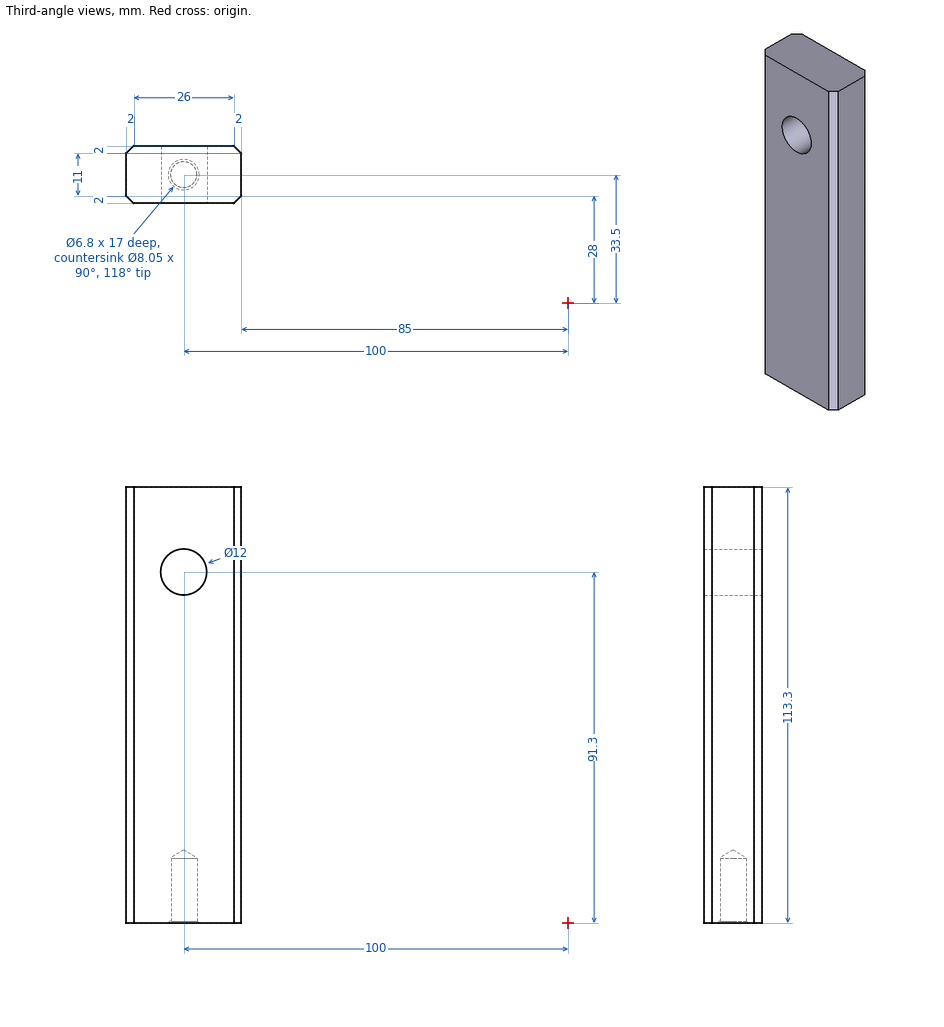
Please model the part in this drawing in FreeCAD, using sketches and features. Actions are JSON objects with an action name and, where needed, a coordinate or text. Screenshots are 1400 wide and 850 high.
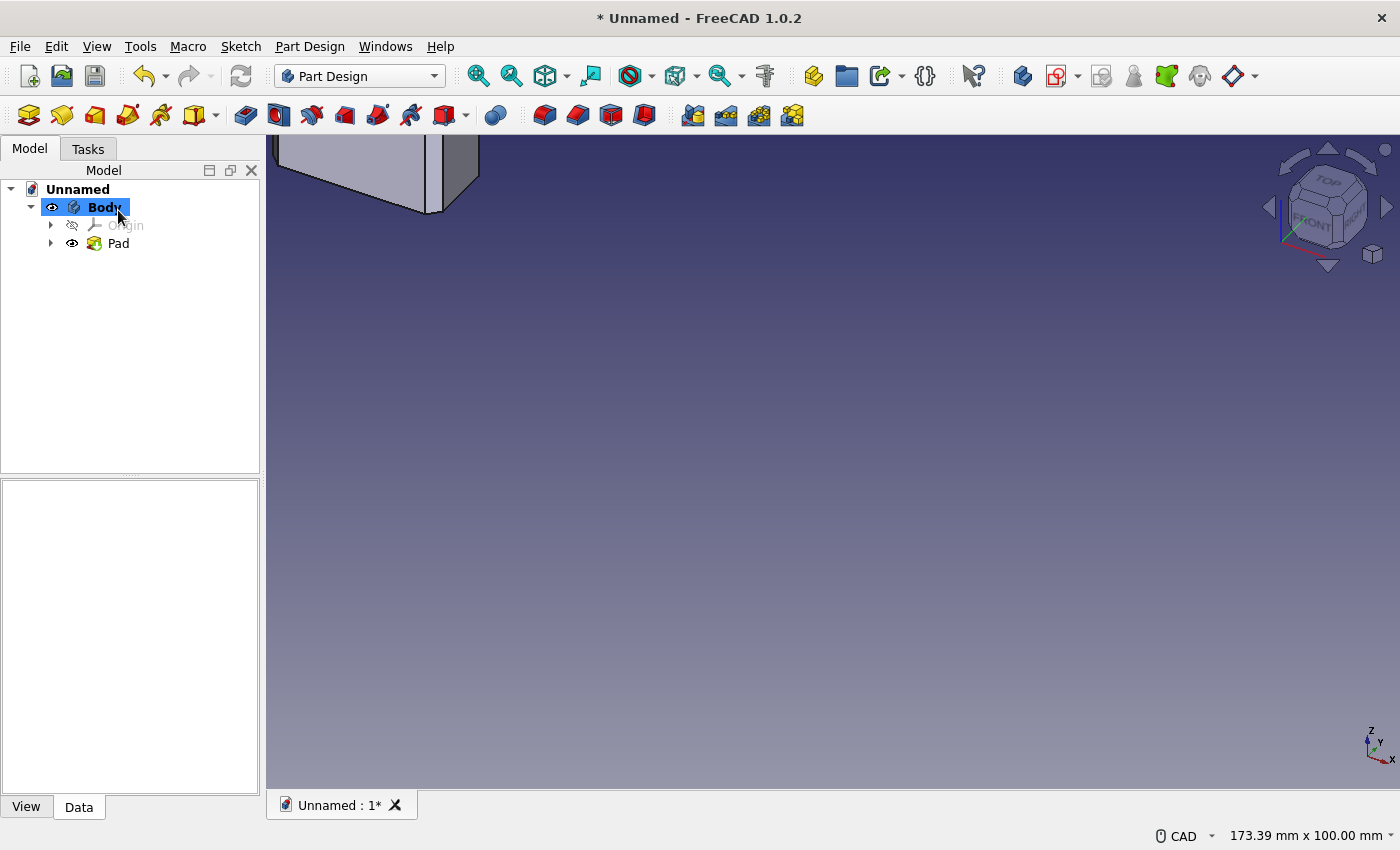
{"action": "left_click", "coordinate": [479, 76]}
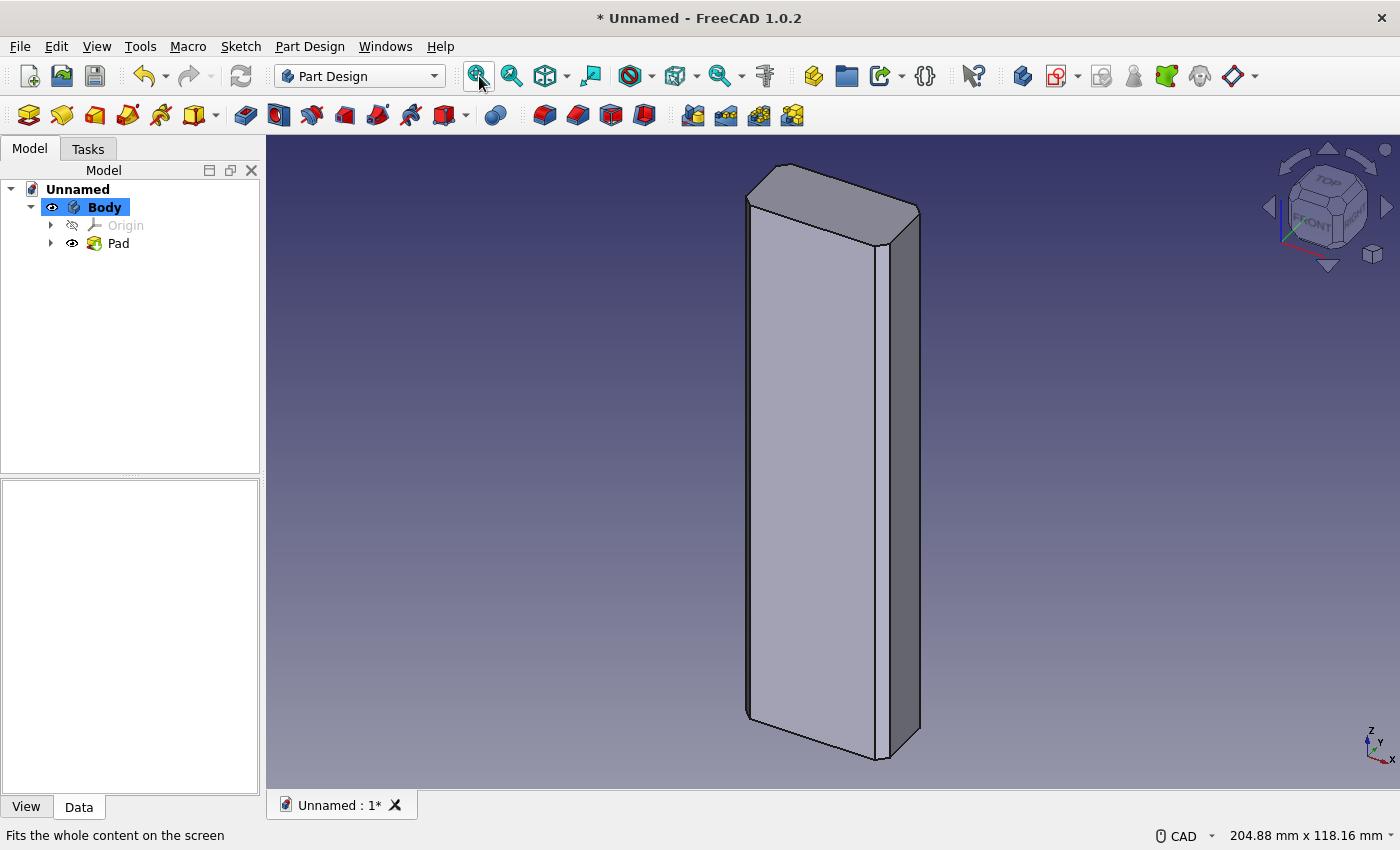
{"action": "left_click", "coordinate": [812, 335]}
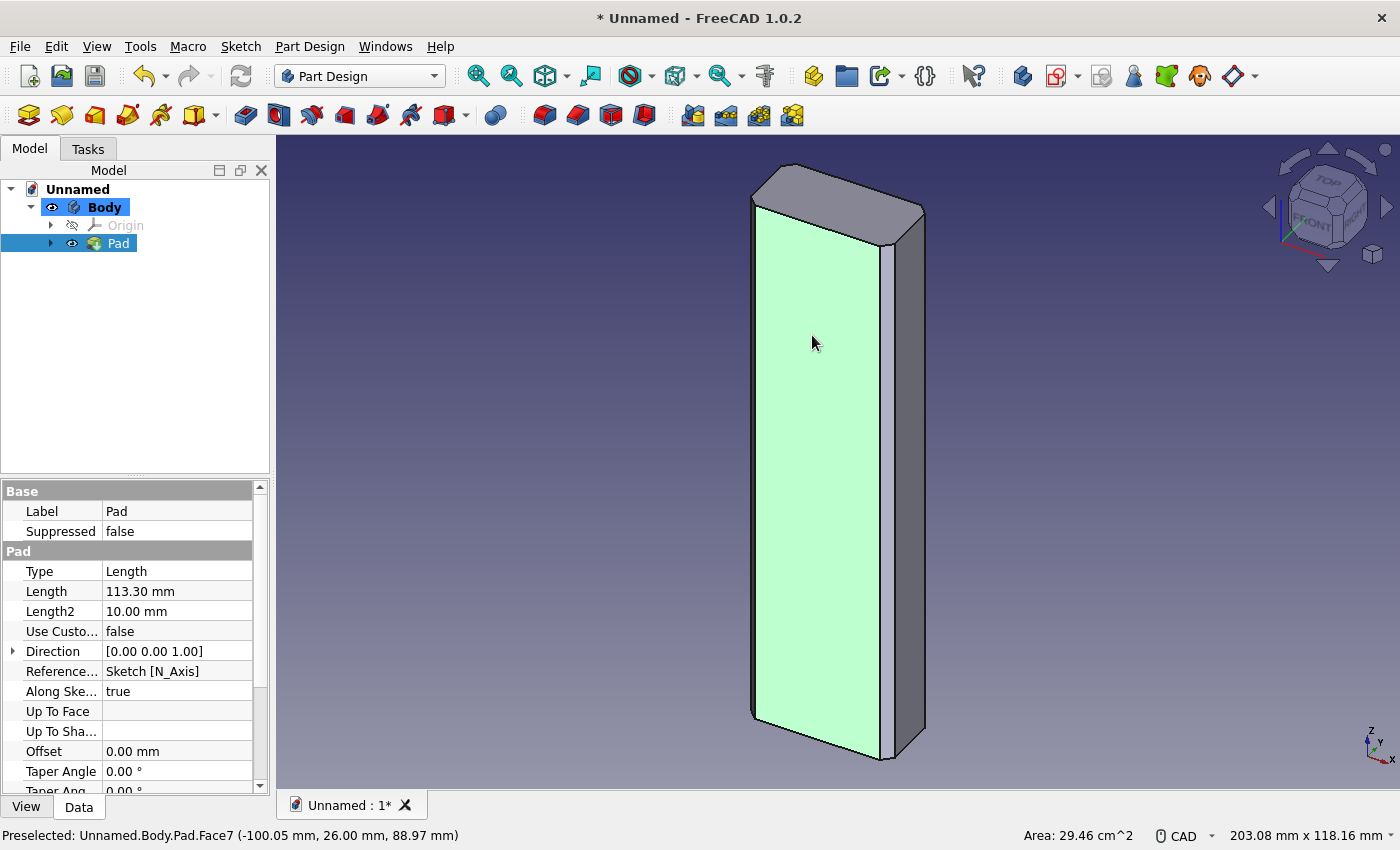
{"action": "left_click", "coordinate": [1056, 76]}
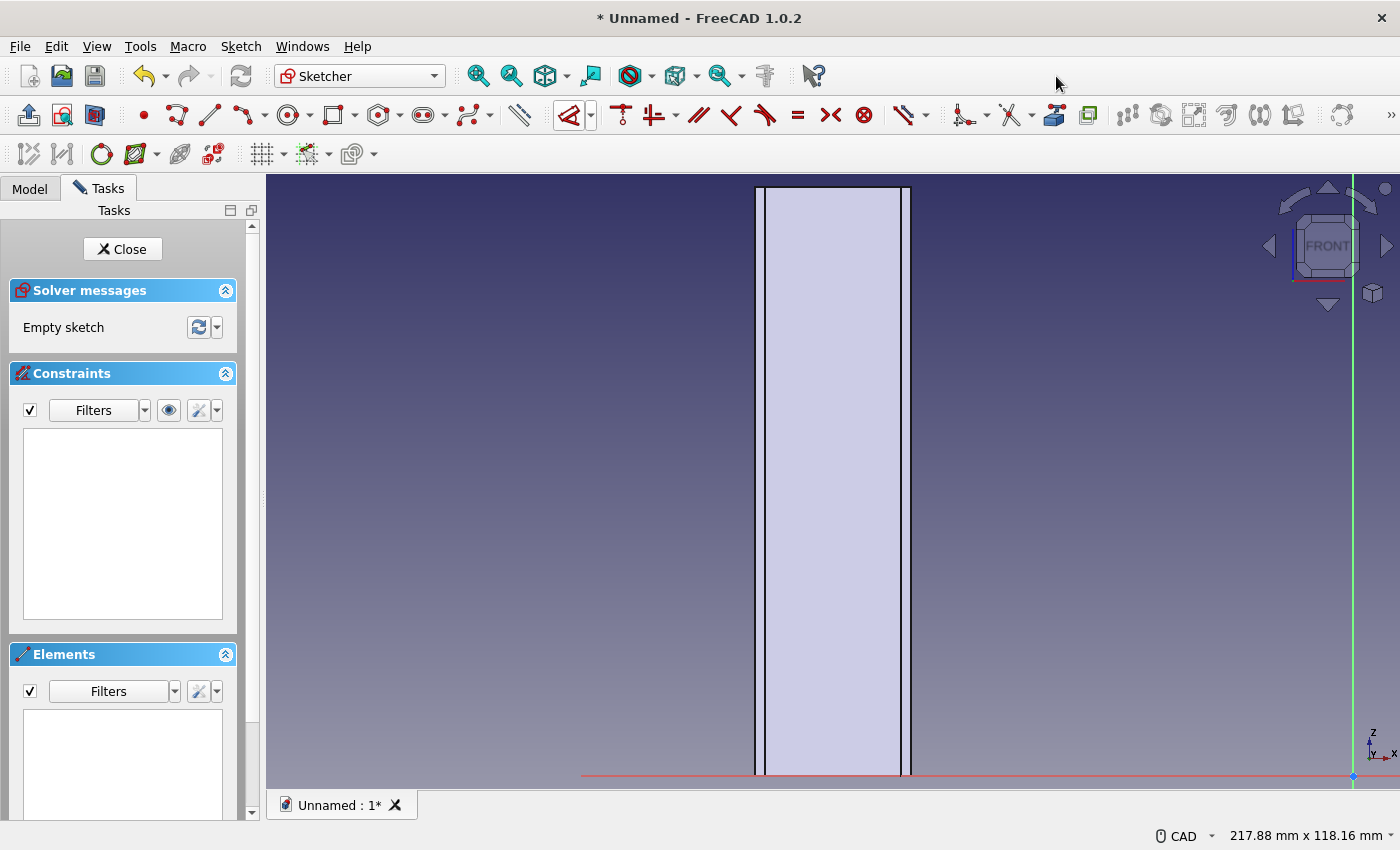
{"action": "scroll", "coordinate": [847, 265], "scroll_direction": "up", "scroll_amount": 9}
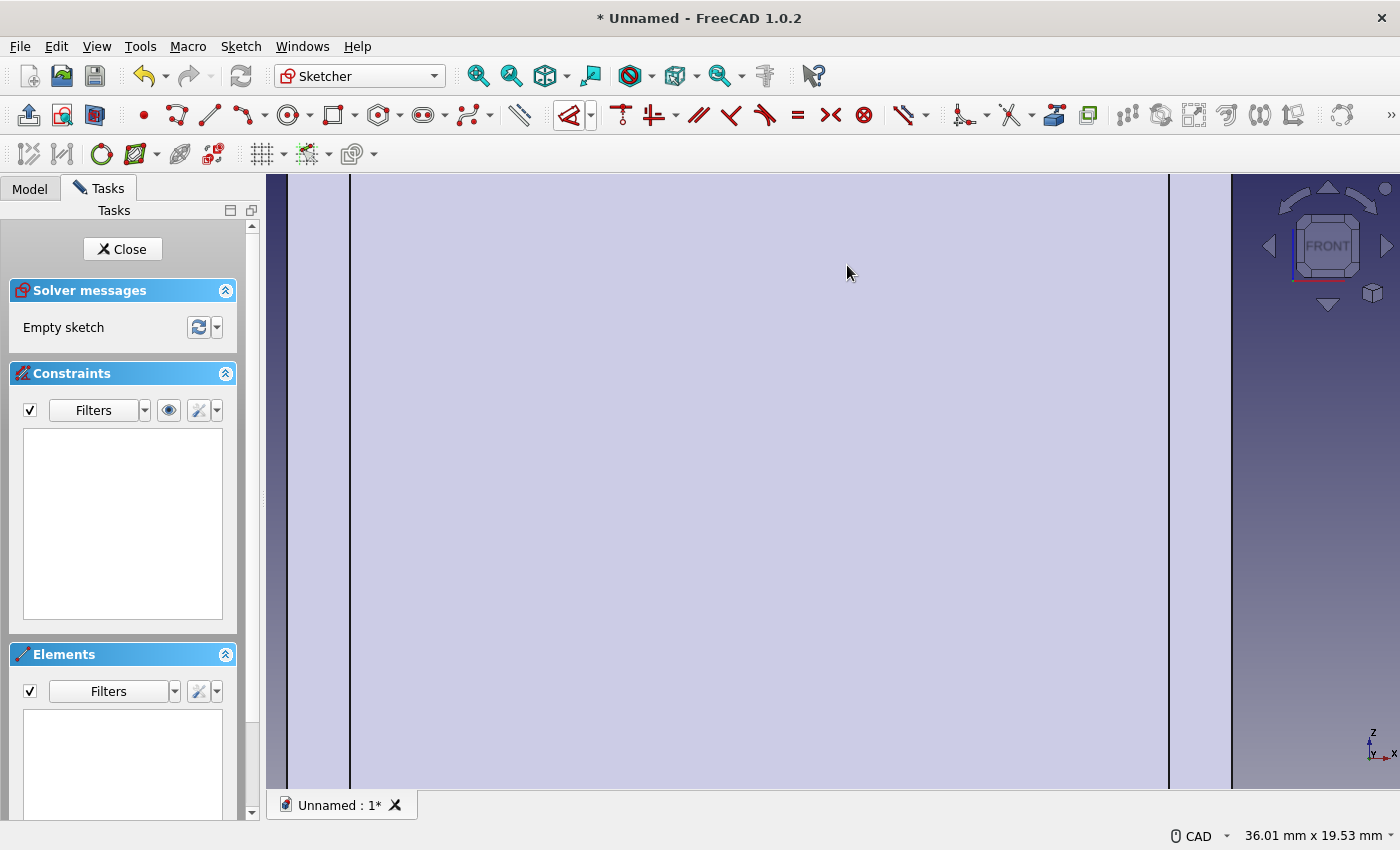
{"action": "left_click", "coordinate": [288, 116]}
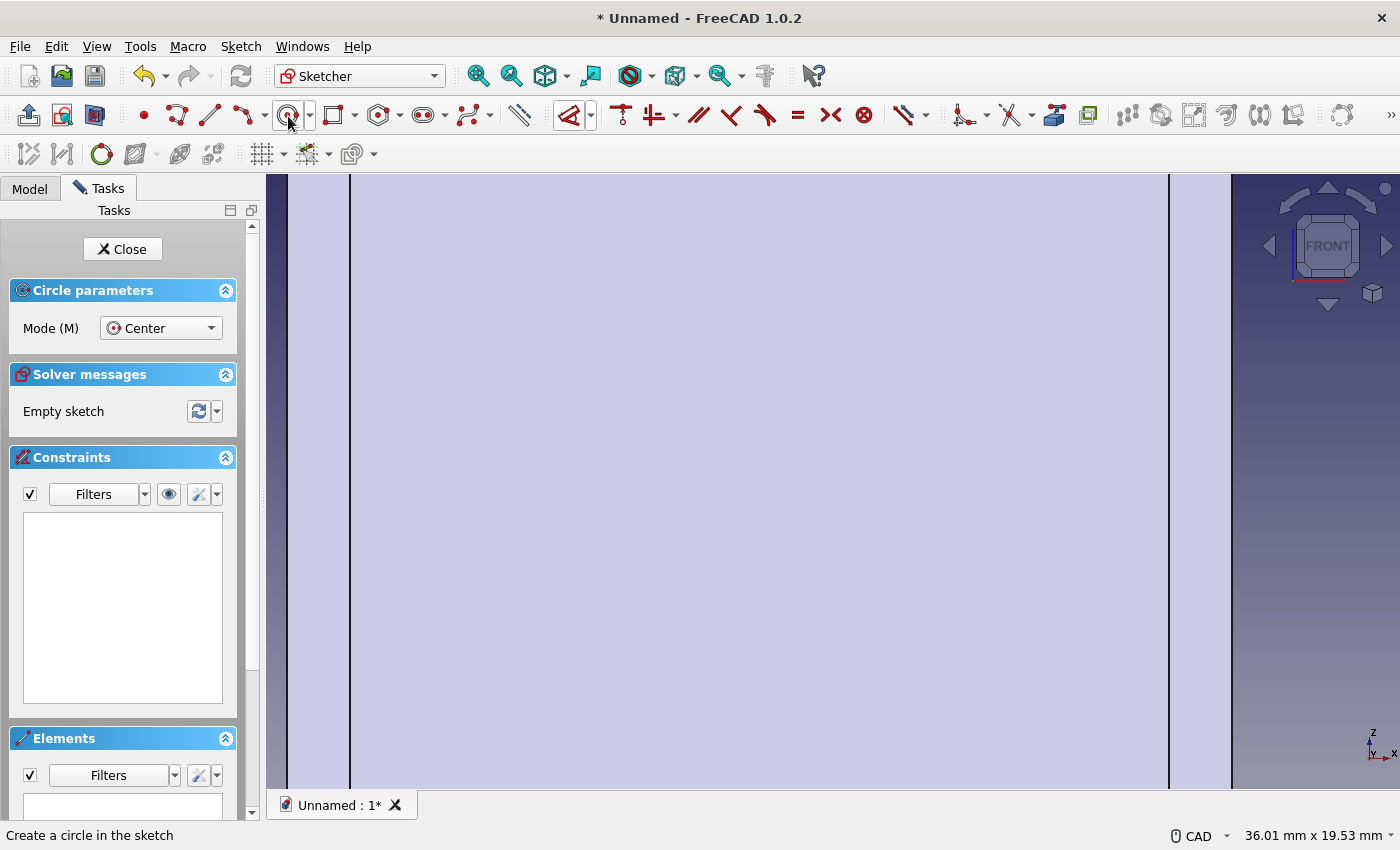
{"action": "left_click", "coordinate": [760, 483]}
{"action": "left_click", "coordinate": [893, 349]}
{"action": "key", "text": "Escape"}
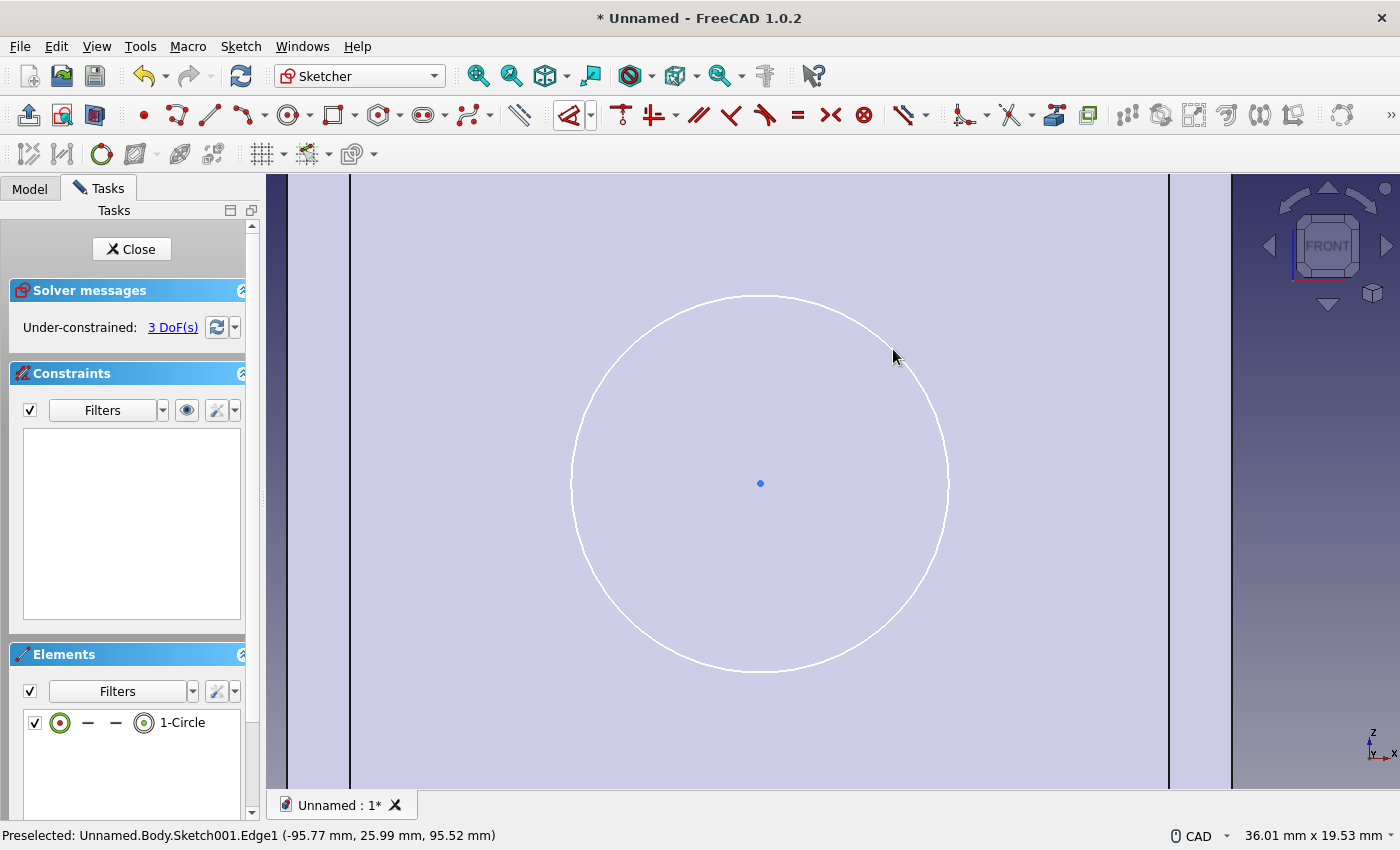
{"action": "left_click", "coordinate": [893, 350]}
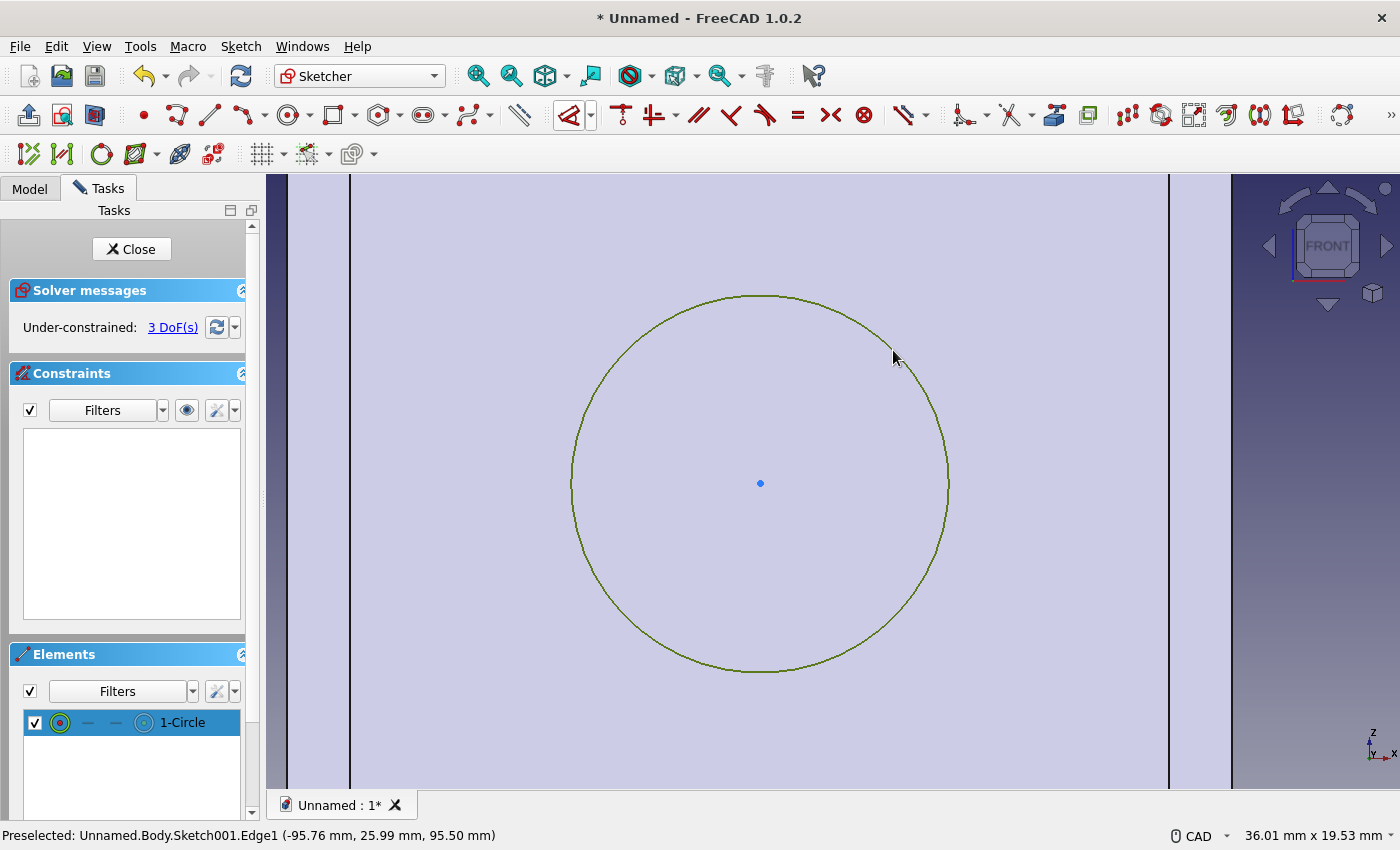
{"action": "left_click", "coordinate": [590, 116]}